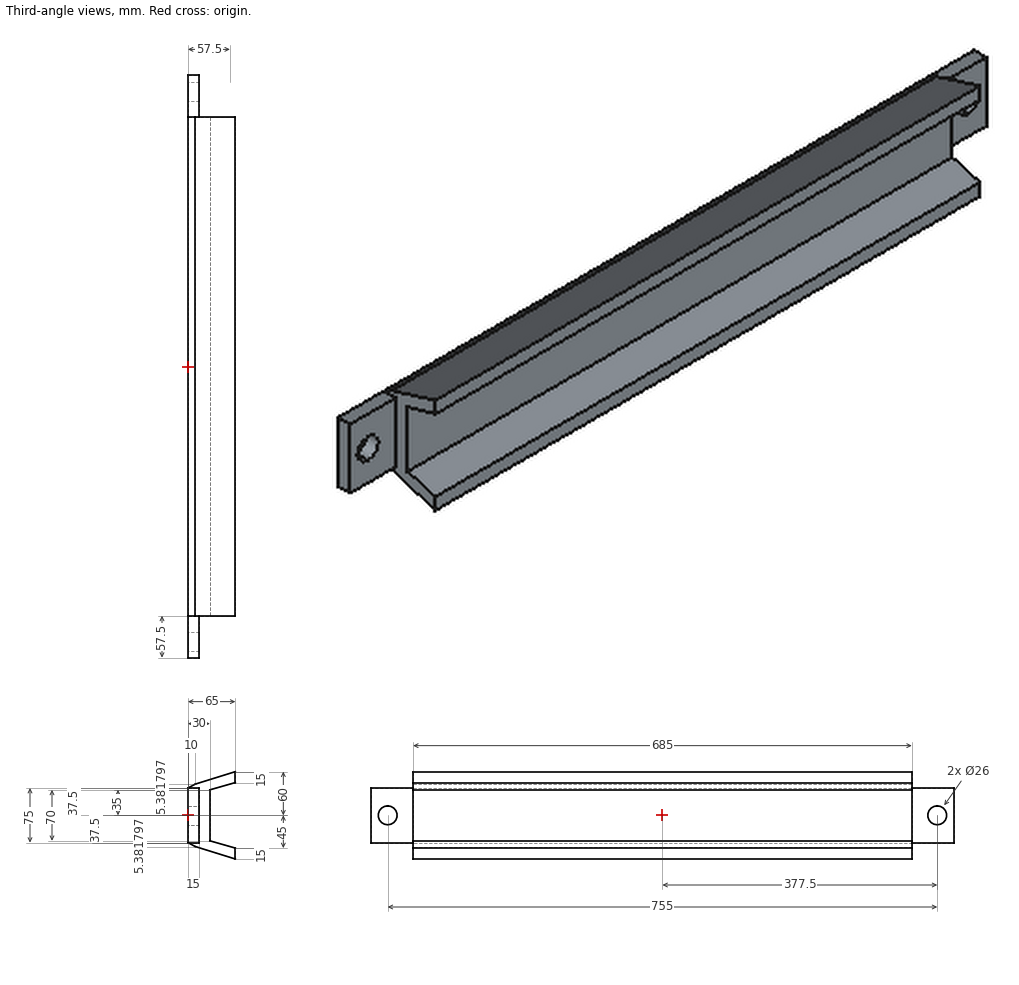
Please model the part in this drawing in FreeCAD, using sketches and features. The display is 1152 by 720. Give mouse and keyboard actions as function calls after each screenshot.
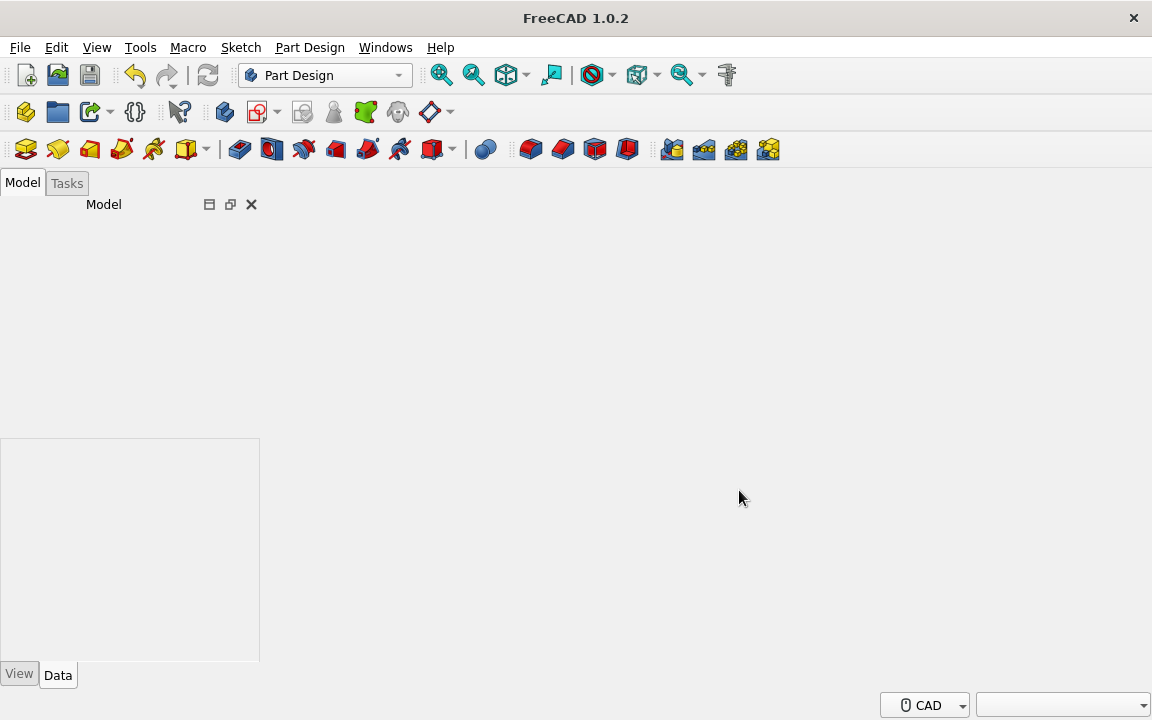
click(26, 76)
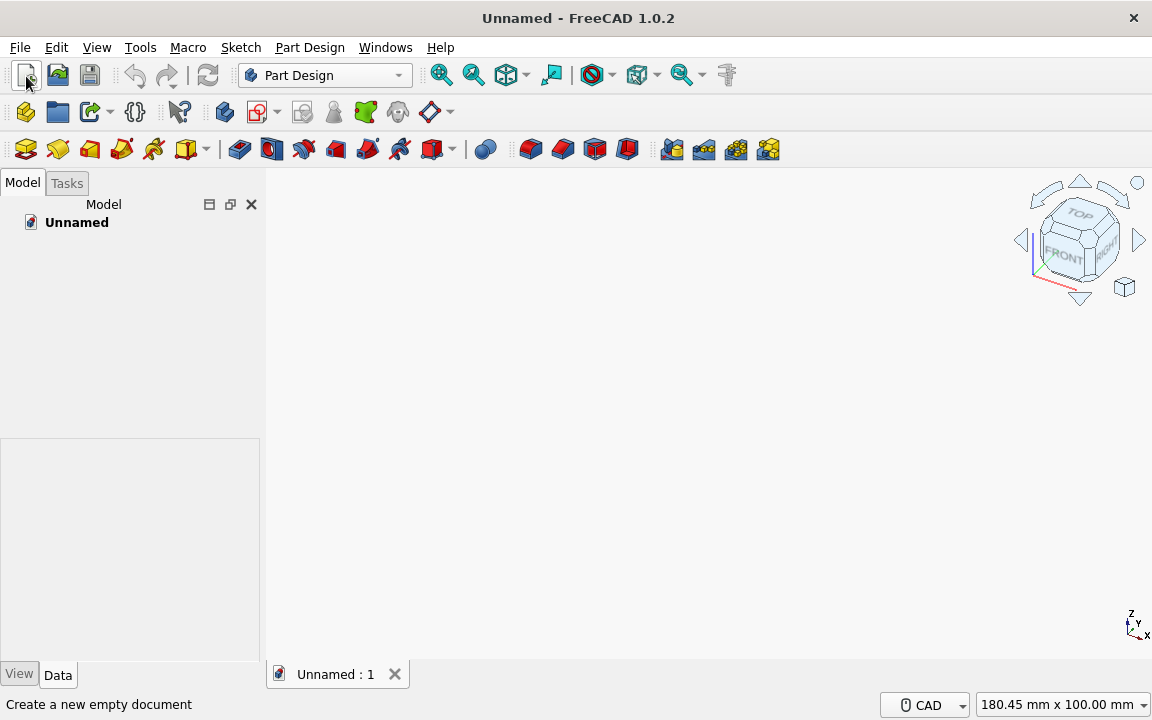
click(258, 112)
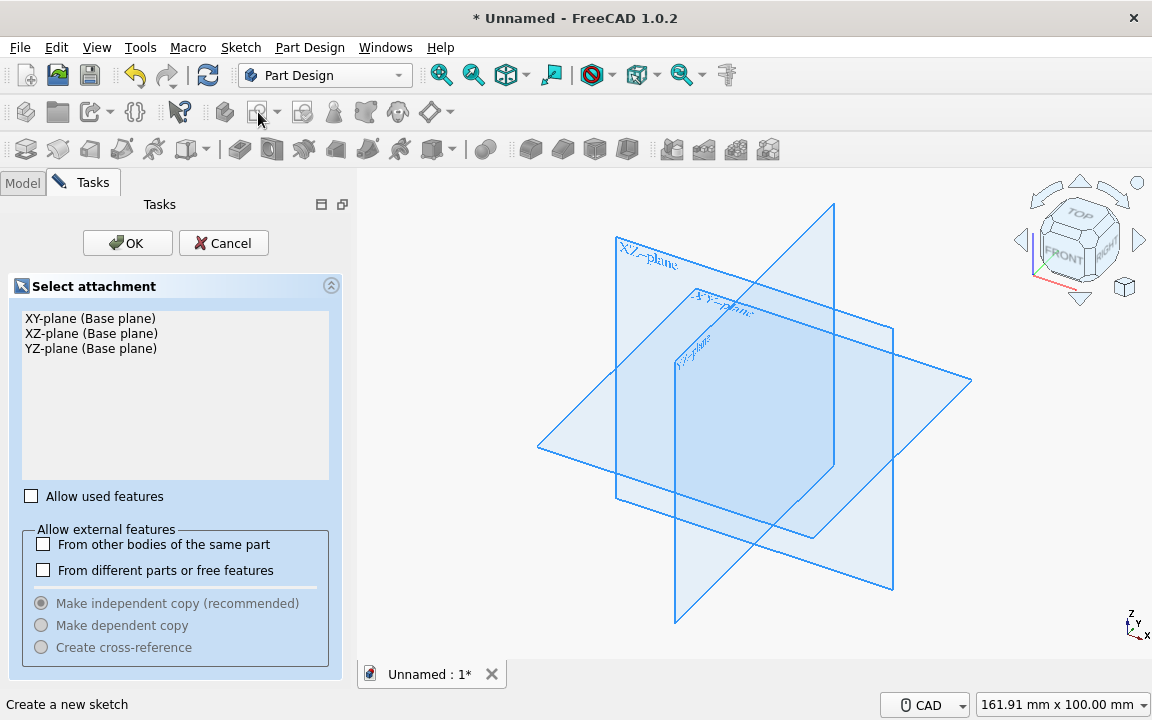
click(82, 334)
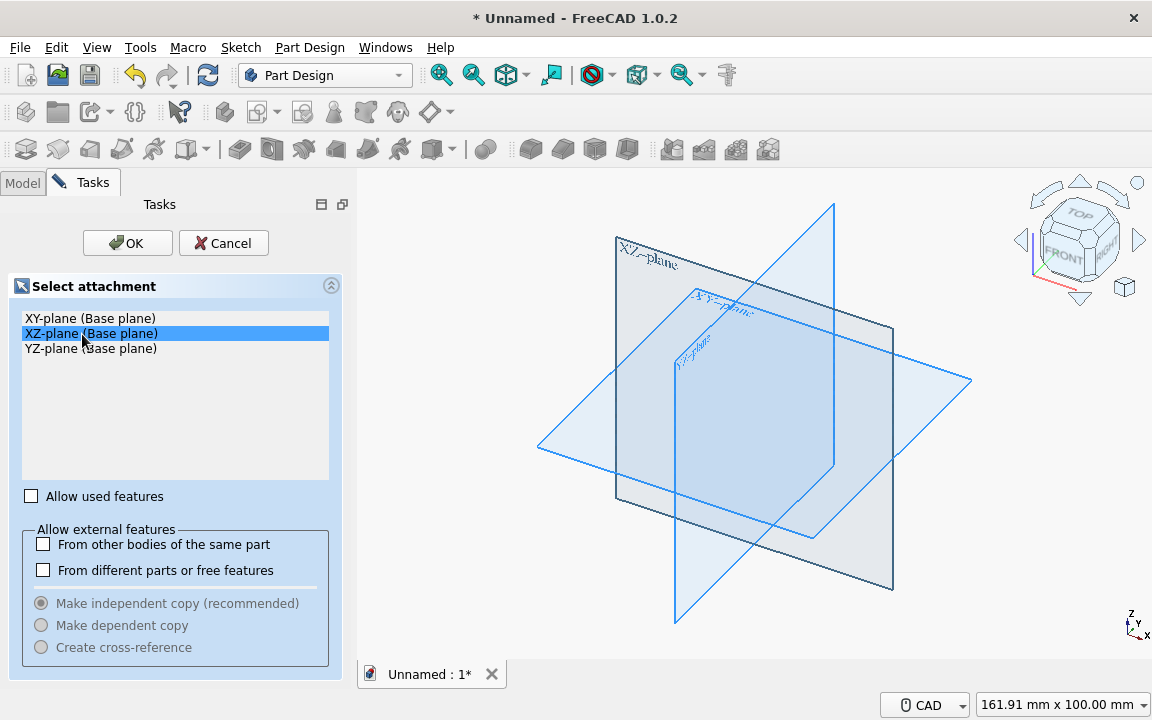
click(128, 243)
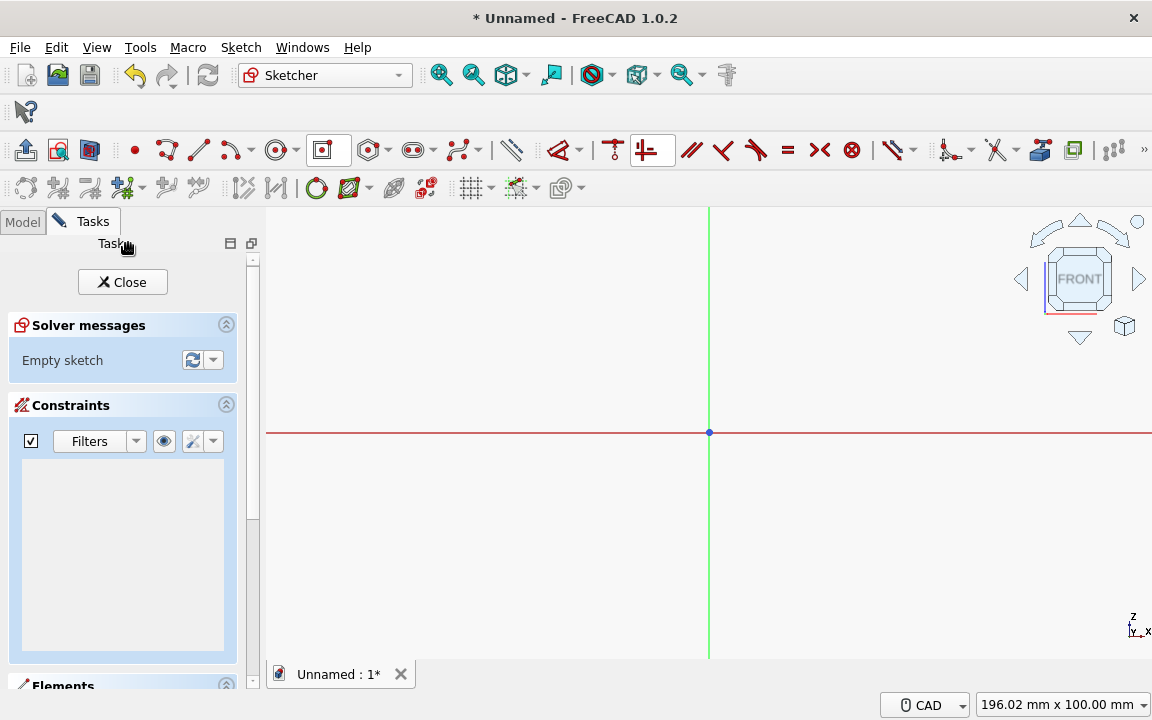
scroll(378, 433, down, 3)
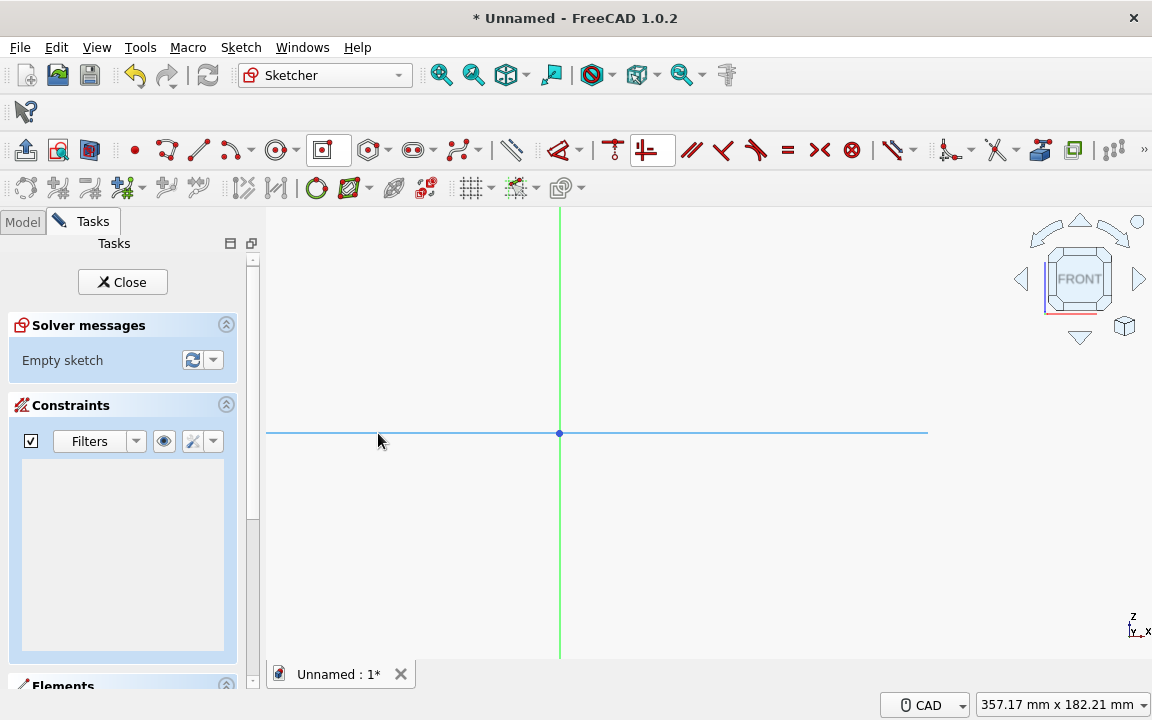
click(168, 150)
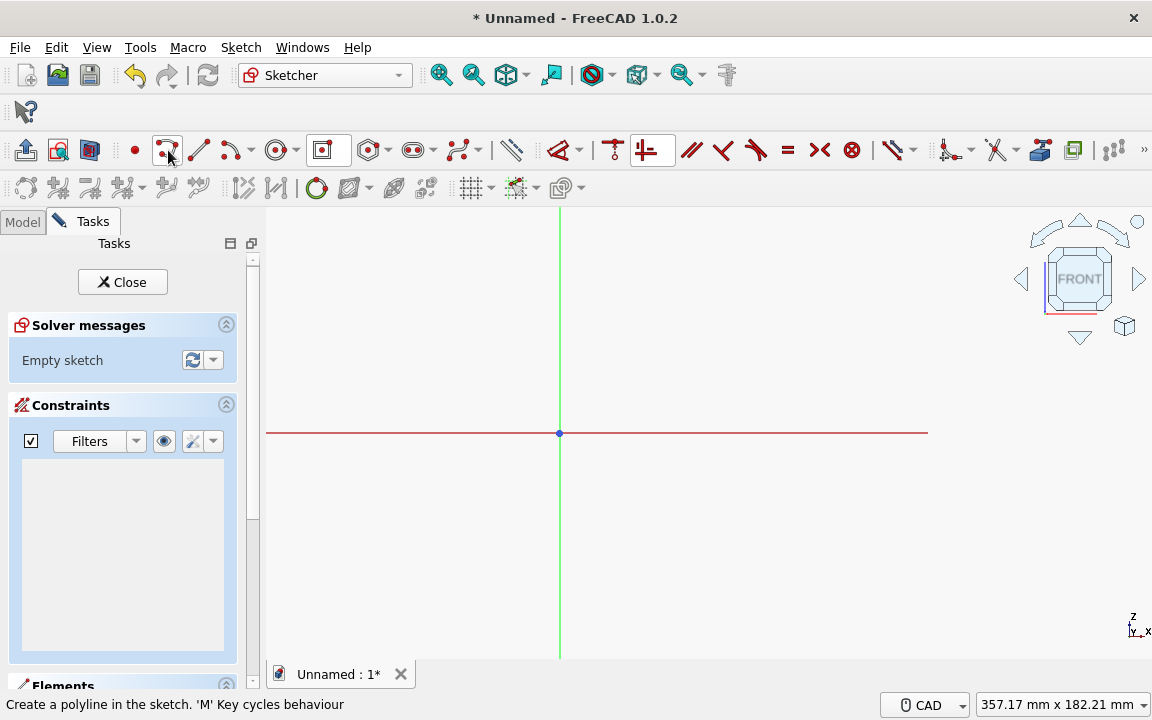
click(560, 526)
click(569, 340)
click(585, 327)
click(721, 284)
click(721, 322)
click(634, 346)
click(634, 520)
click(721, 545)
click(721, 582)
click(585, 540)
click(560, 527)
key(Escape)
key(Escape)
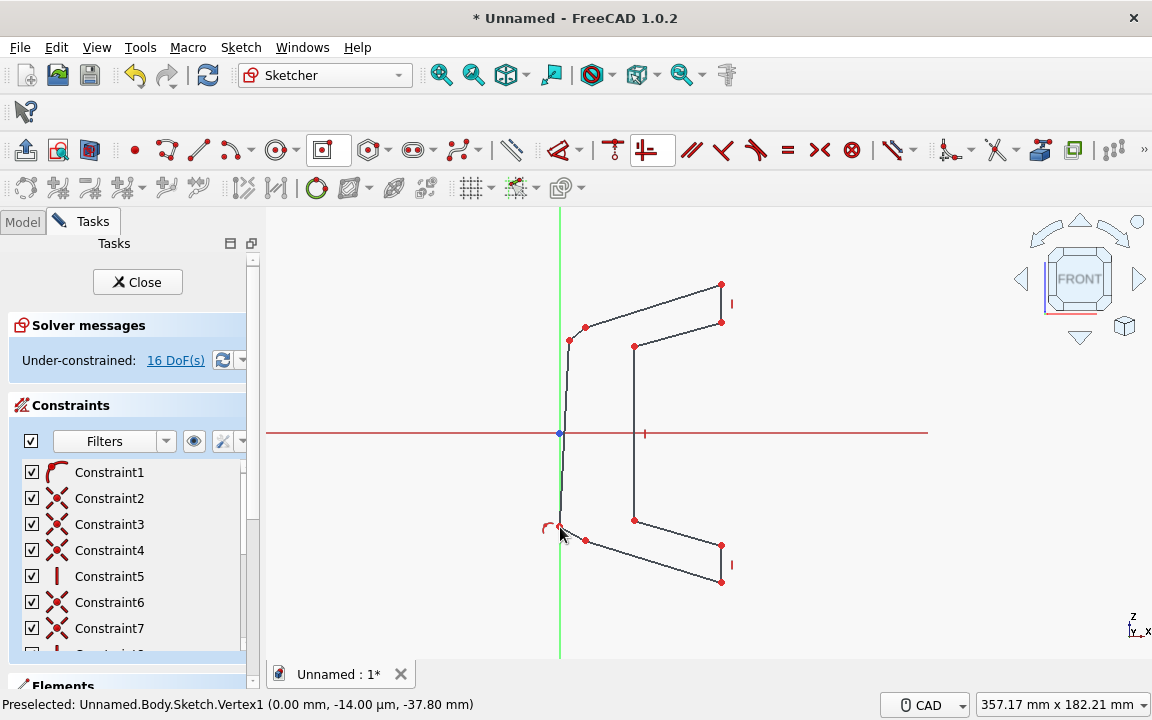
click(562, 471)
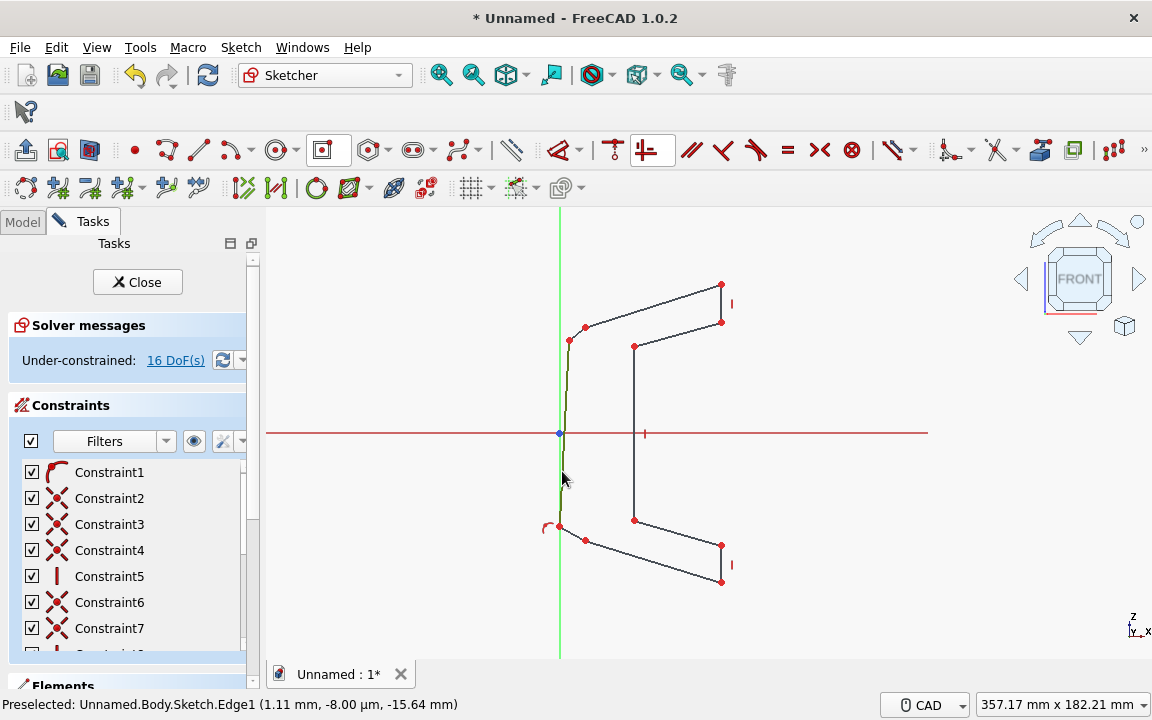
key(v)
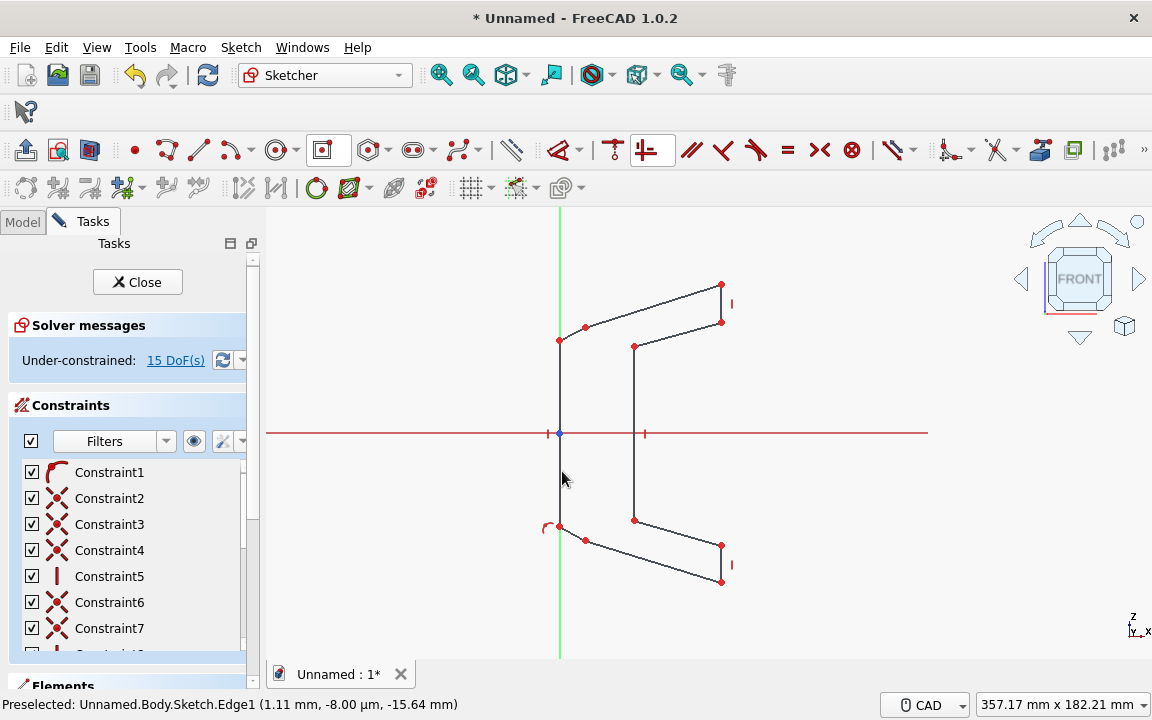
click(558, 150)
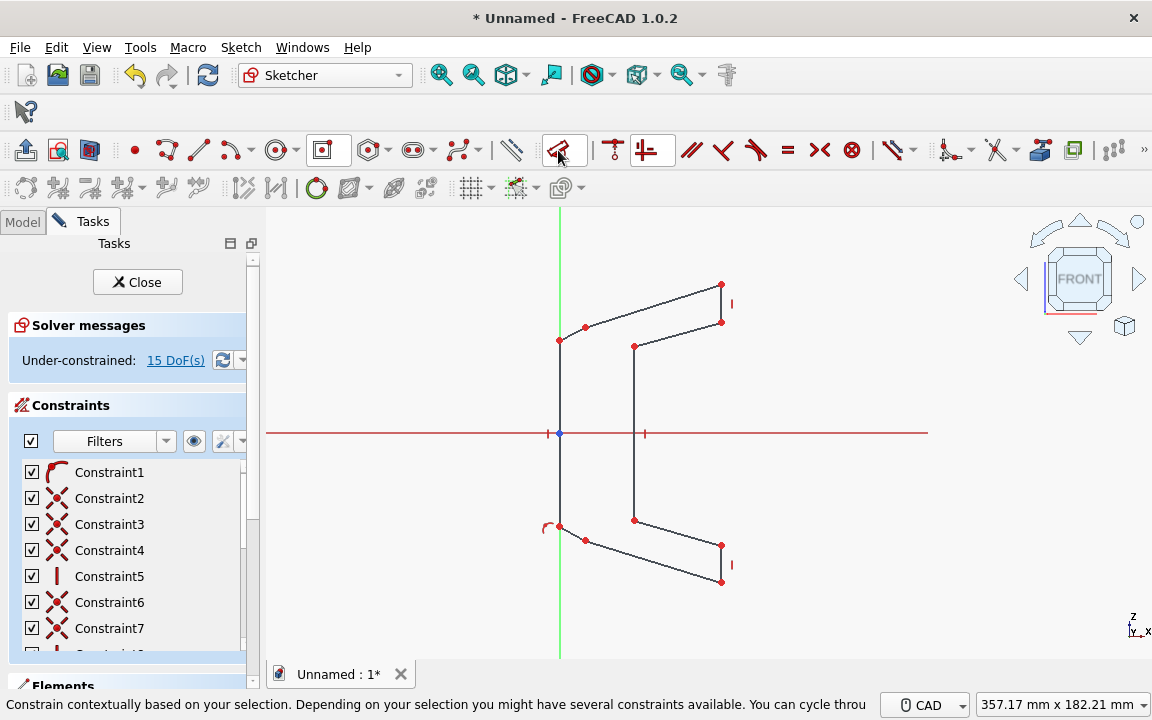
click(560, 471)
click(526, 391)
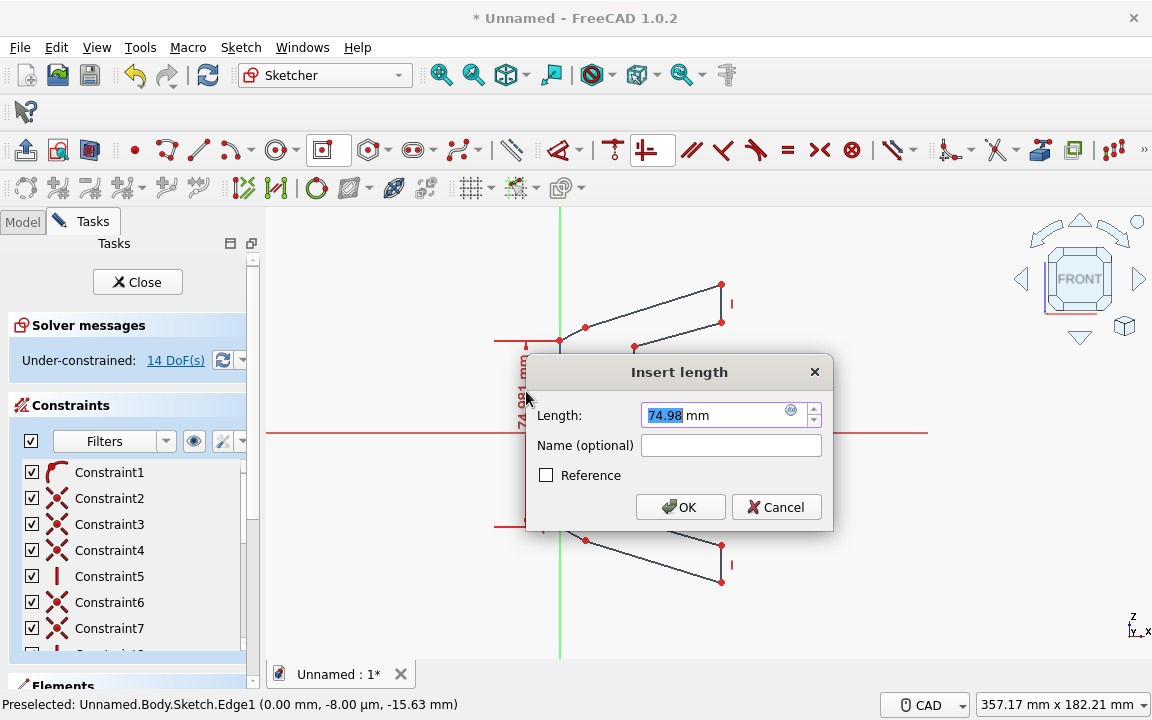
text(75)
key(Return)